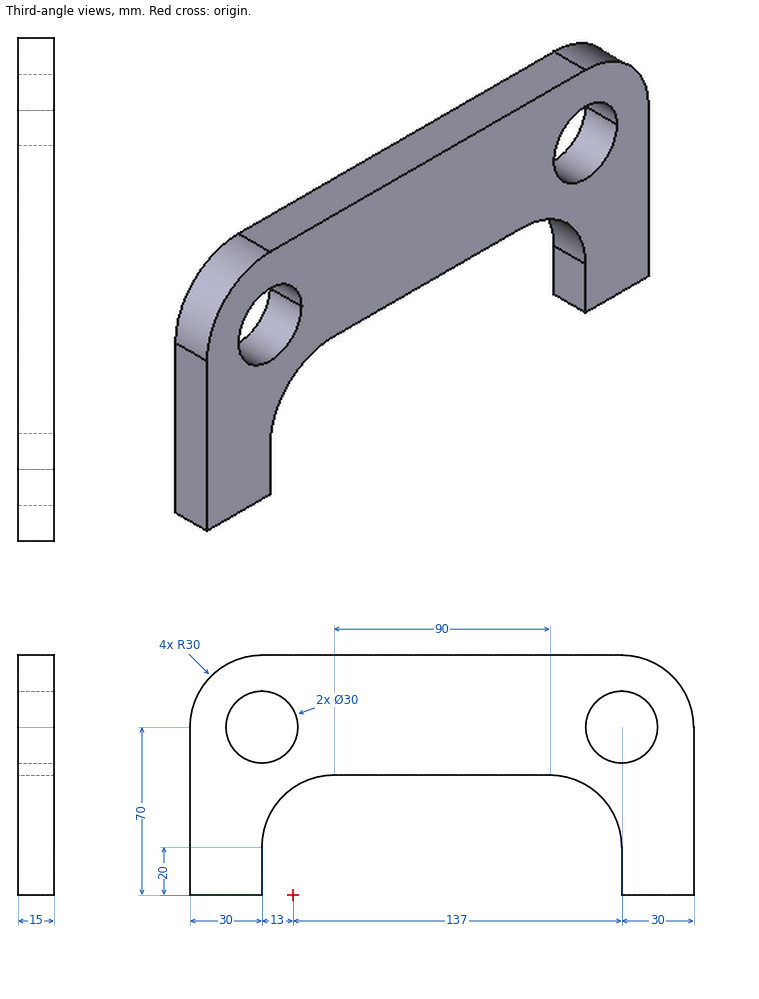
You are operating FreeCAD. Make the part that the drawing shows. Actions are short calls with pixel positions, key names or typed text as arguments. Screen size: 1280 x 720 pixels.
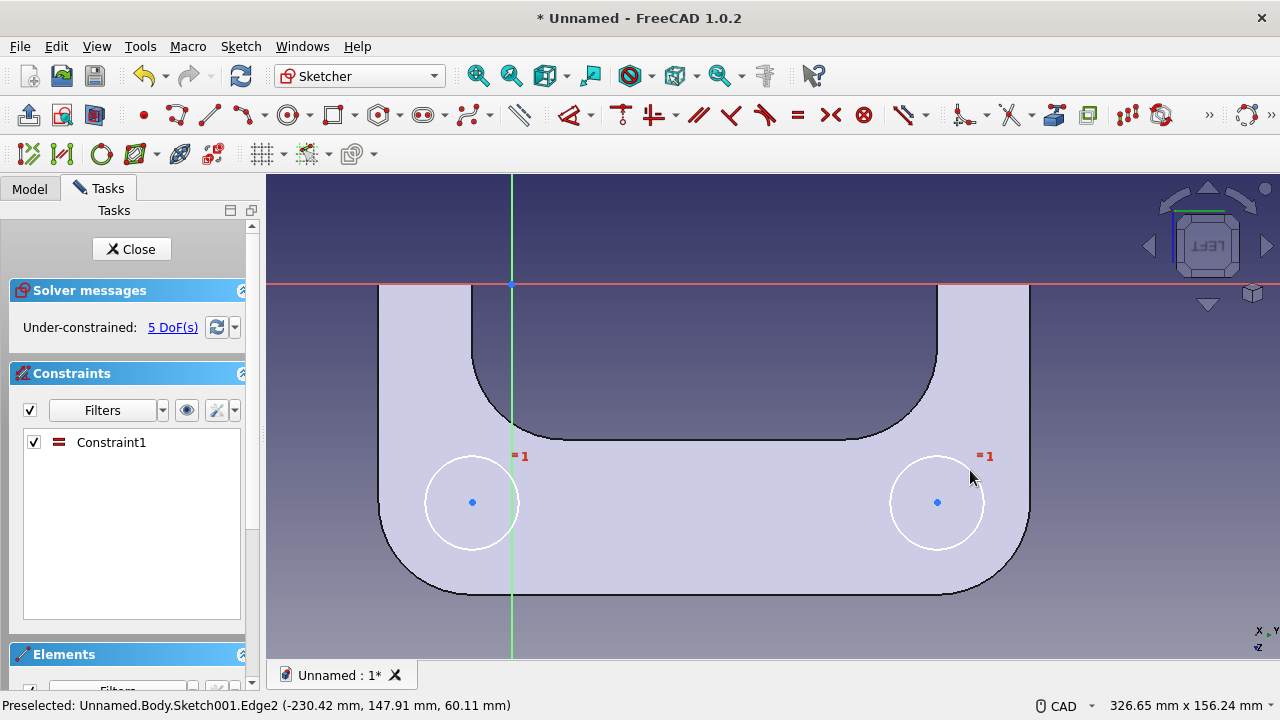
click(472, 503)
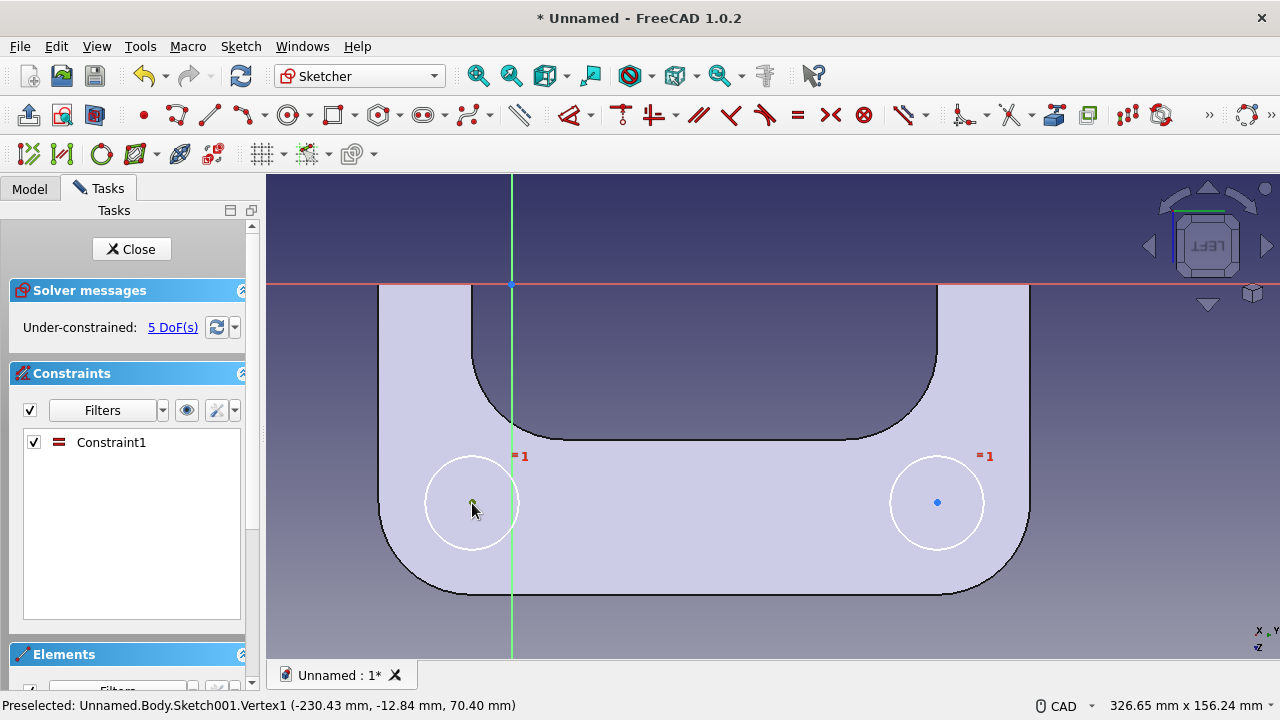
click(937, 503)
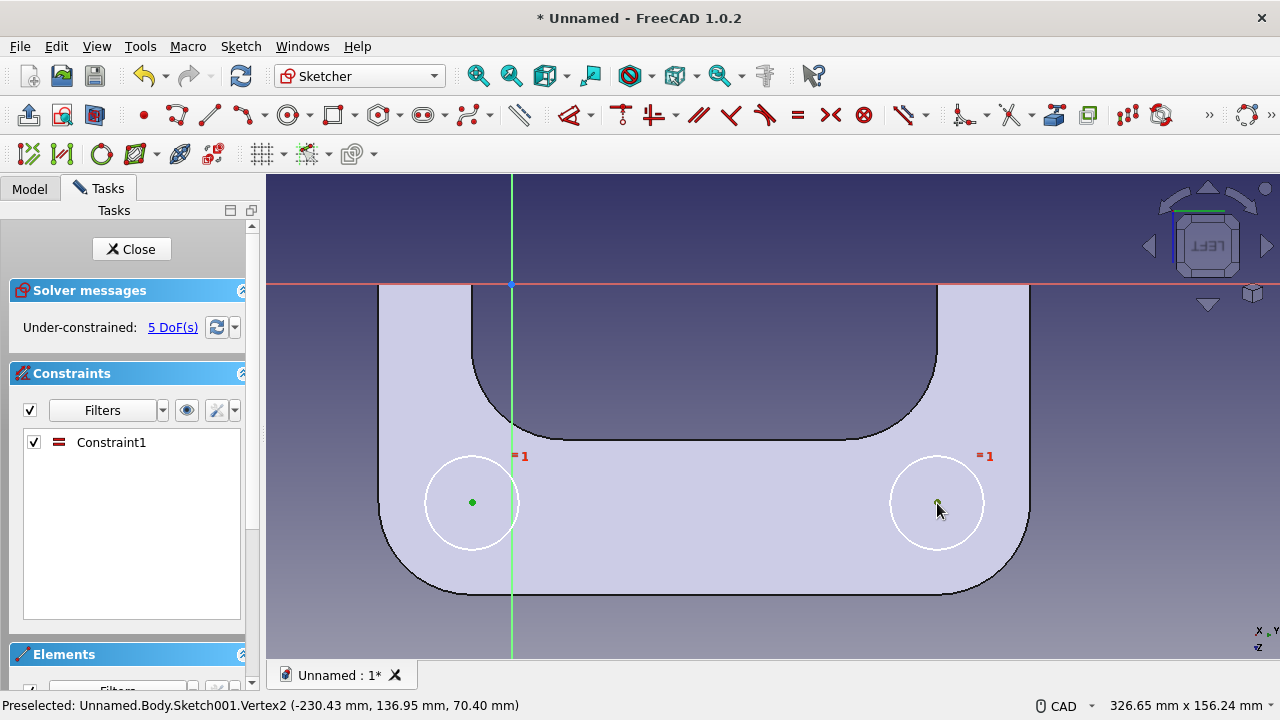
key(h)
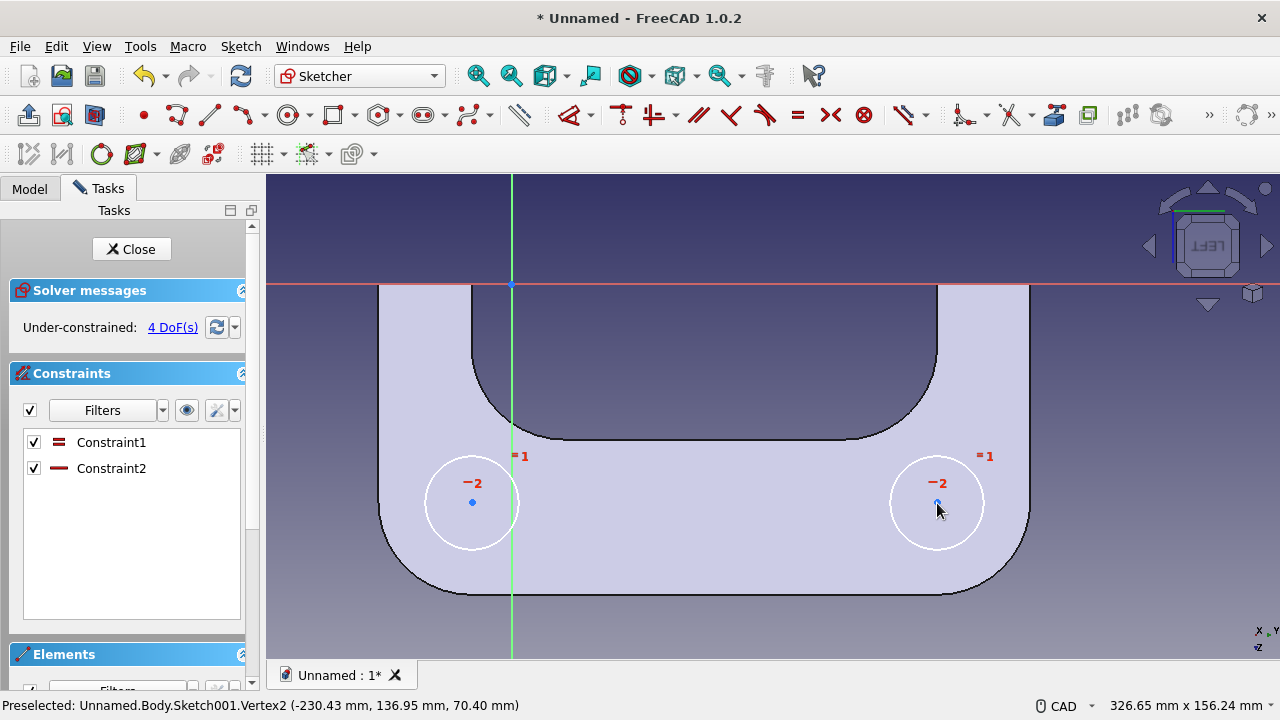
key(d)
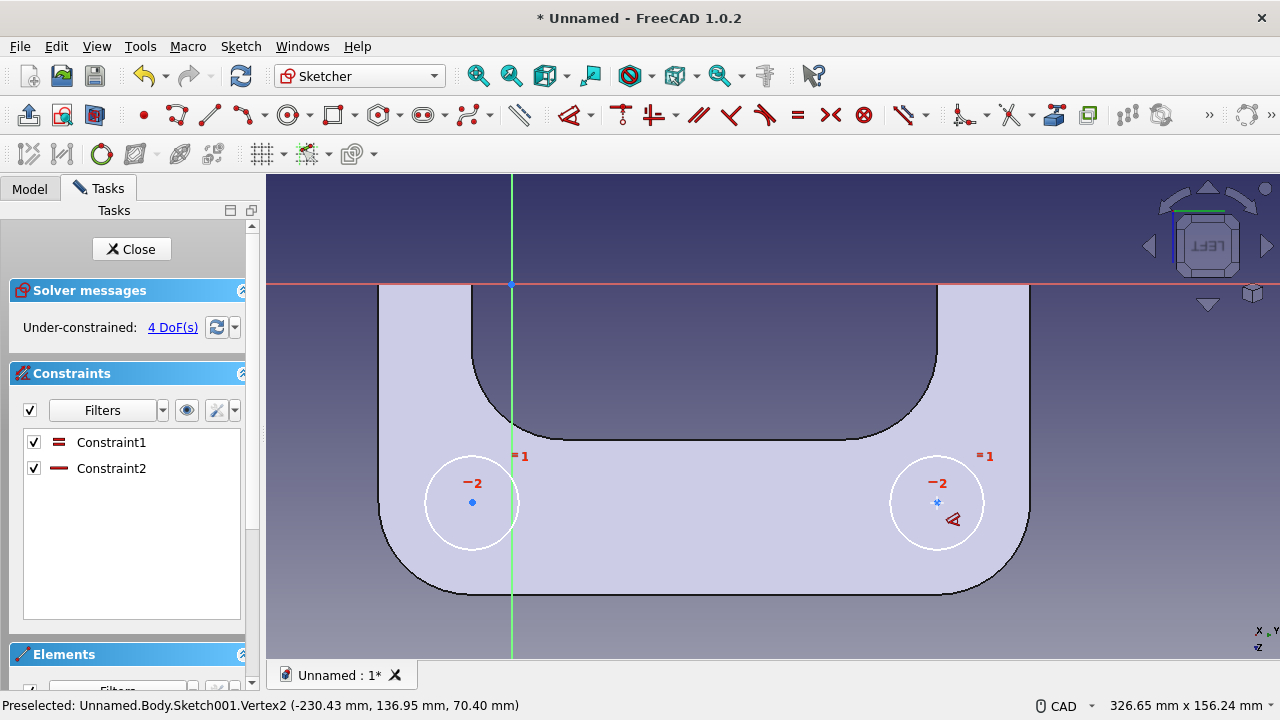
click(439, 470)
click(416, 447)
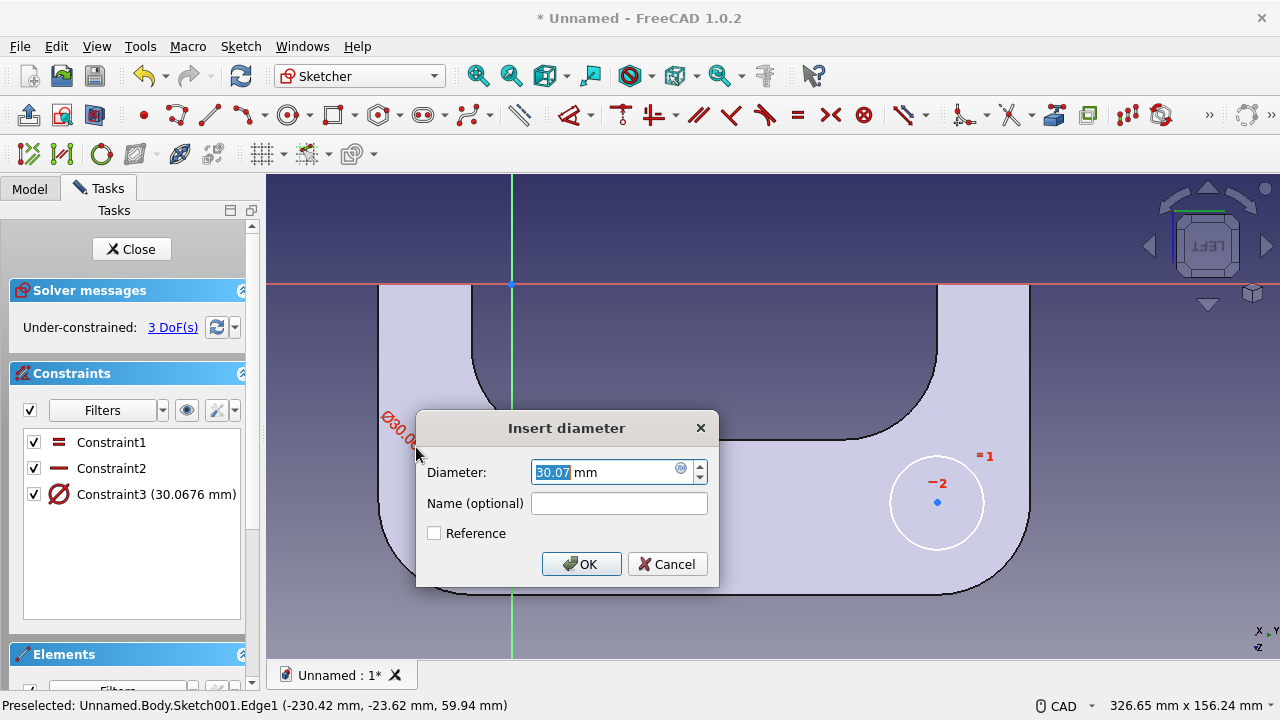
text(30)
key(Return)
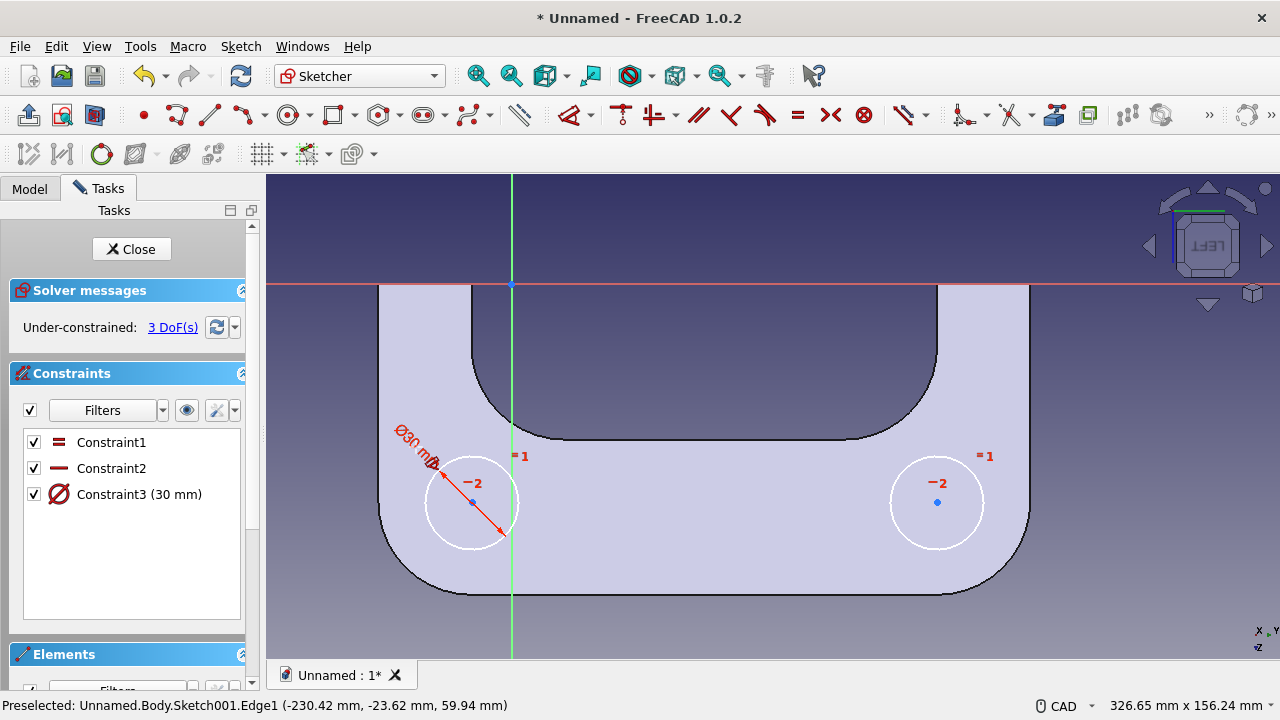
click(472, 503)
click(492, 250)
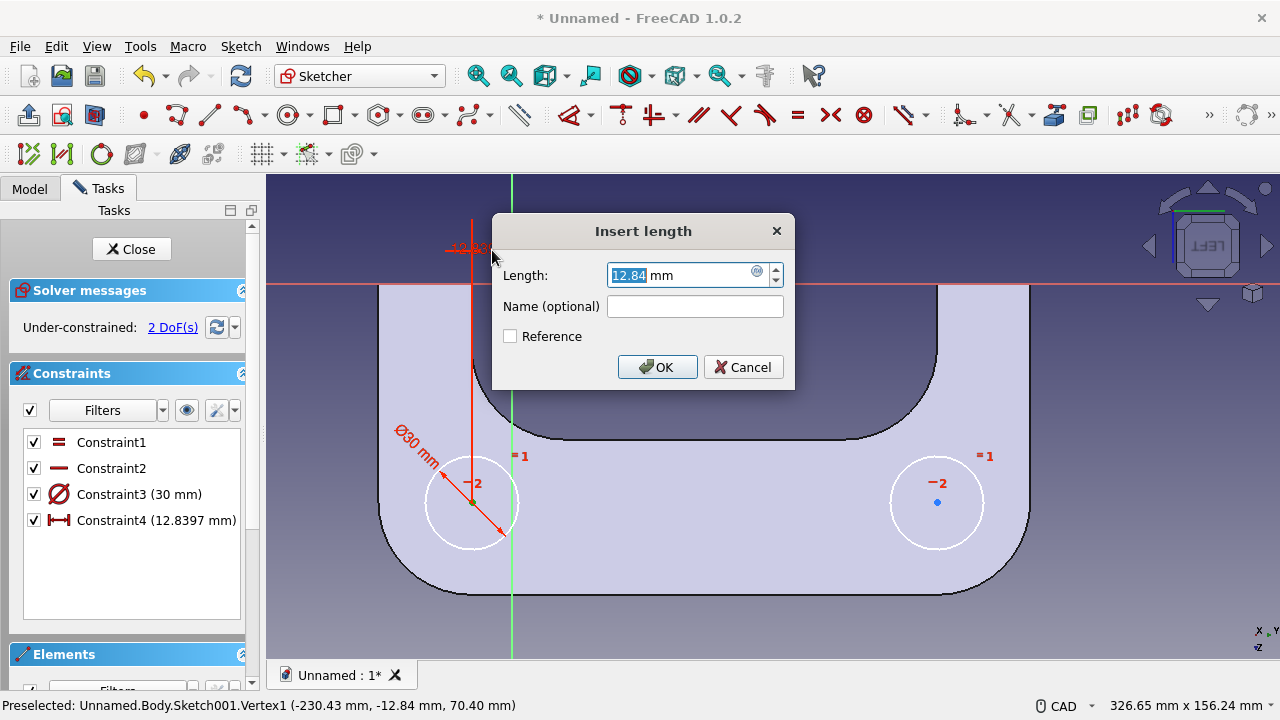
text(13)
key(Return)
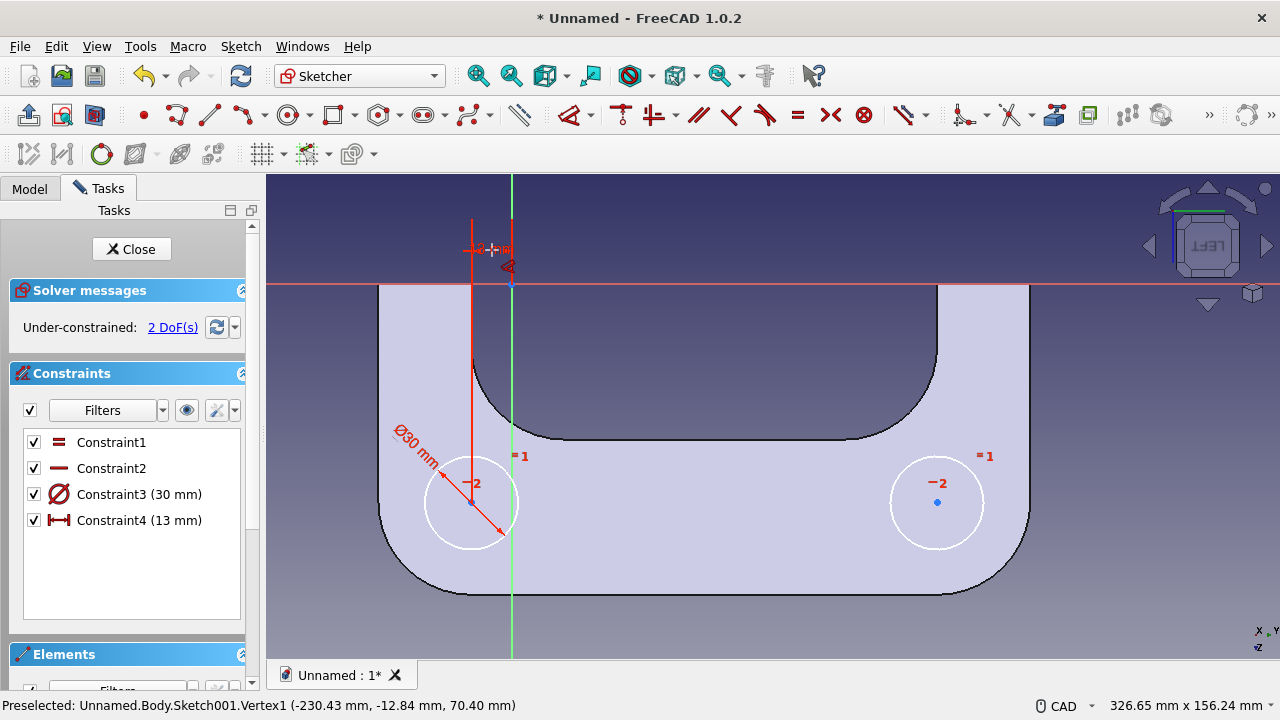
click(472, 503)
click(438, 394)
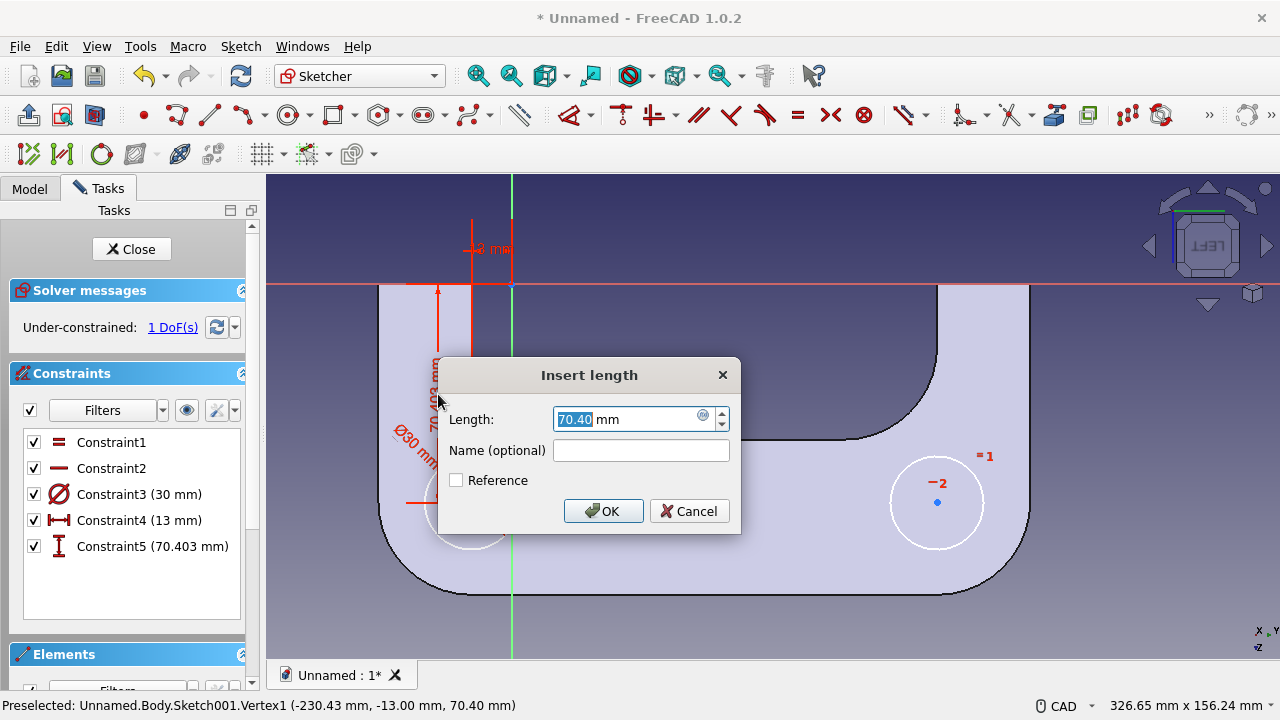
text(70)
key(Return)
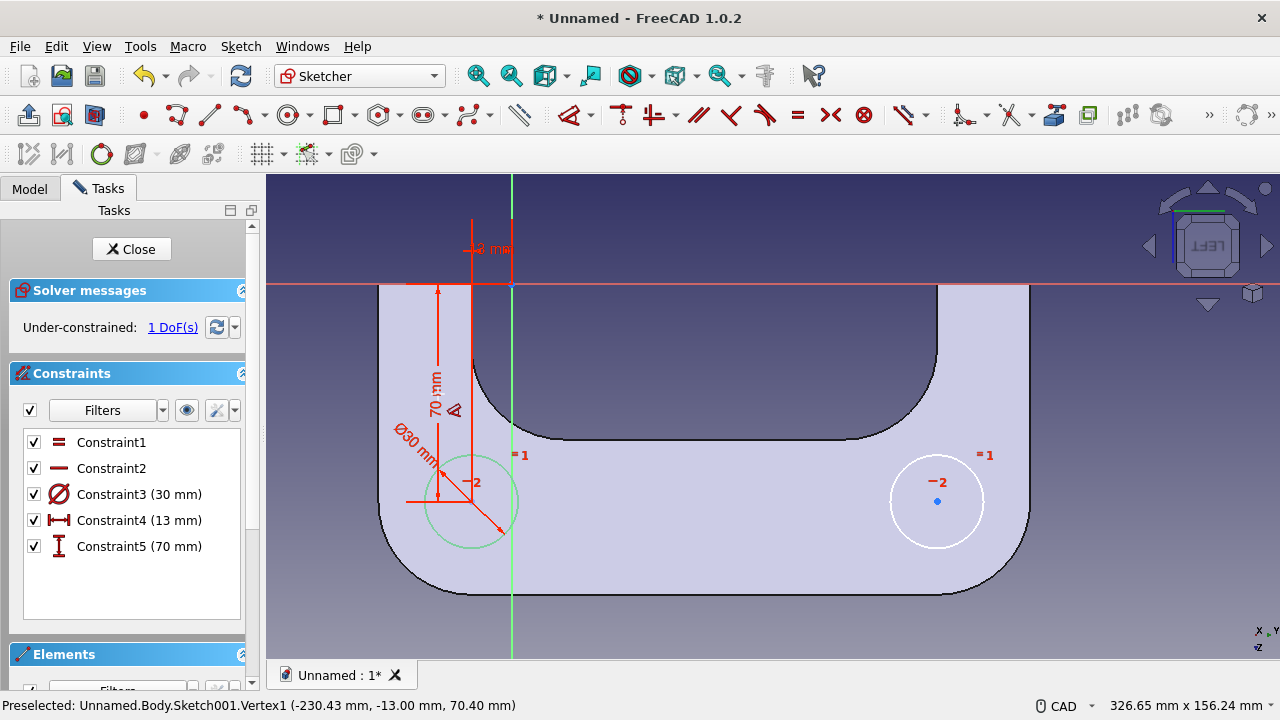
click(937, 502)
click(724, 250)